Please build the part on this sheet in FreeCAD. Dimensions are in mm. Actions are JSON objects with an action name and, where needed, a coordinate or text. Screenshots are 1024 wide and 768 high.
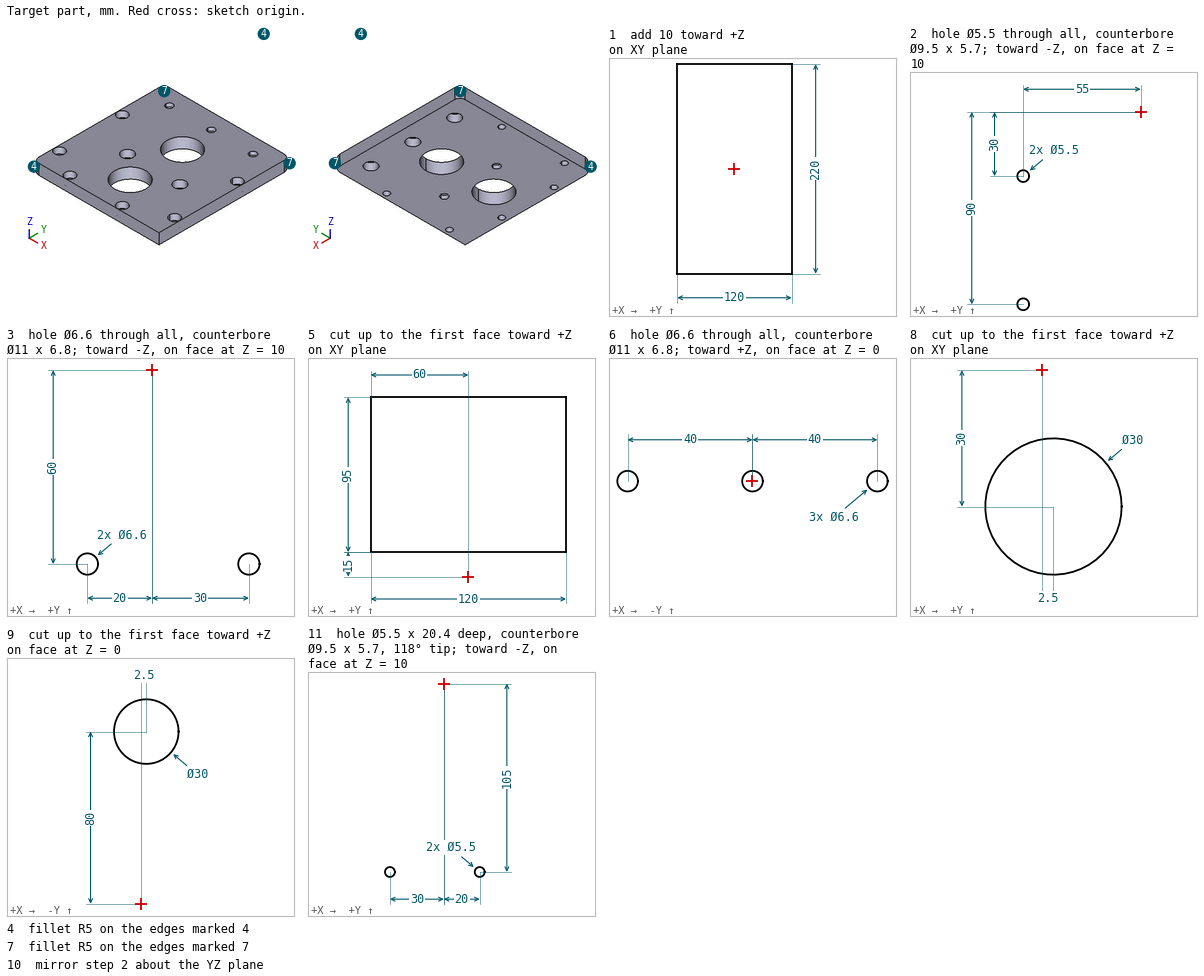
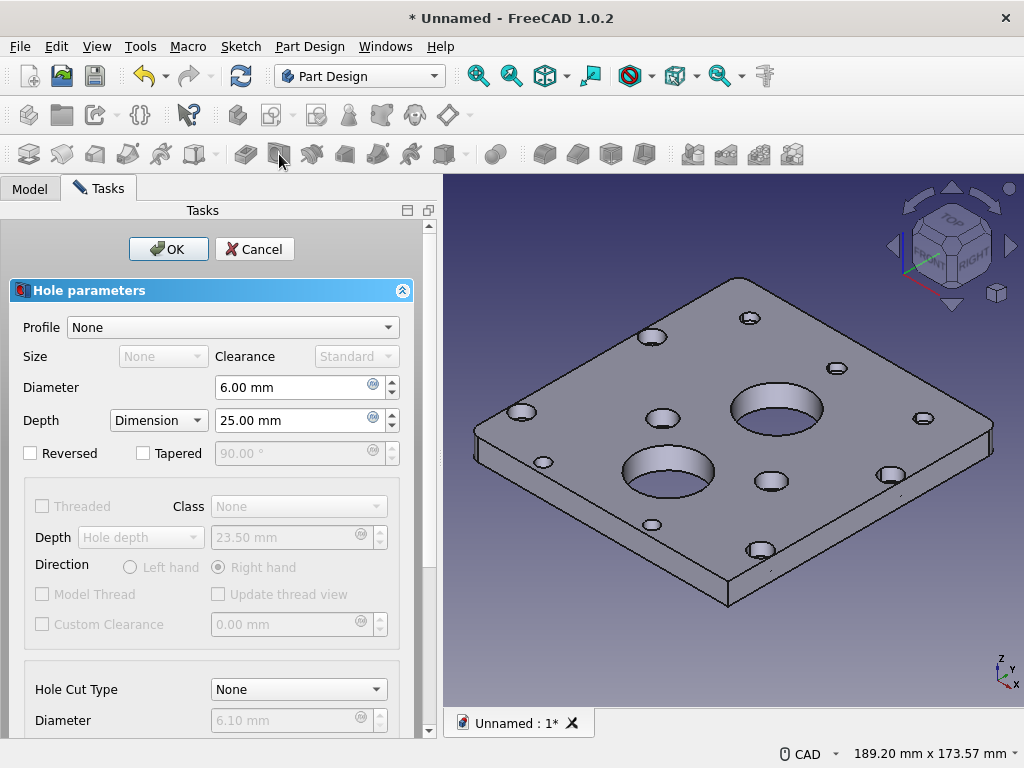
{"action": "triple_click", "coordinate": [300, 388]}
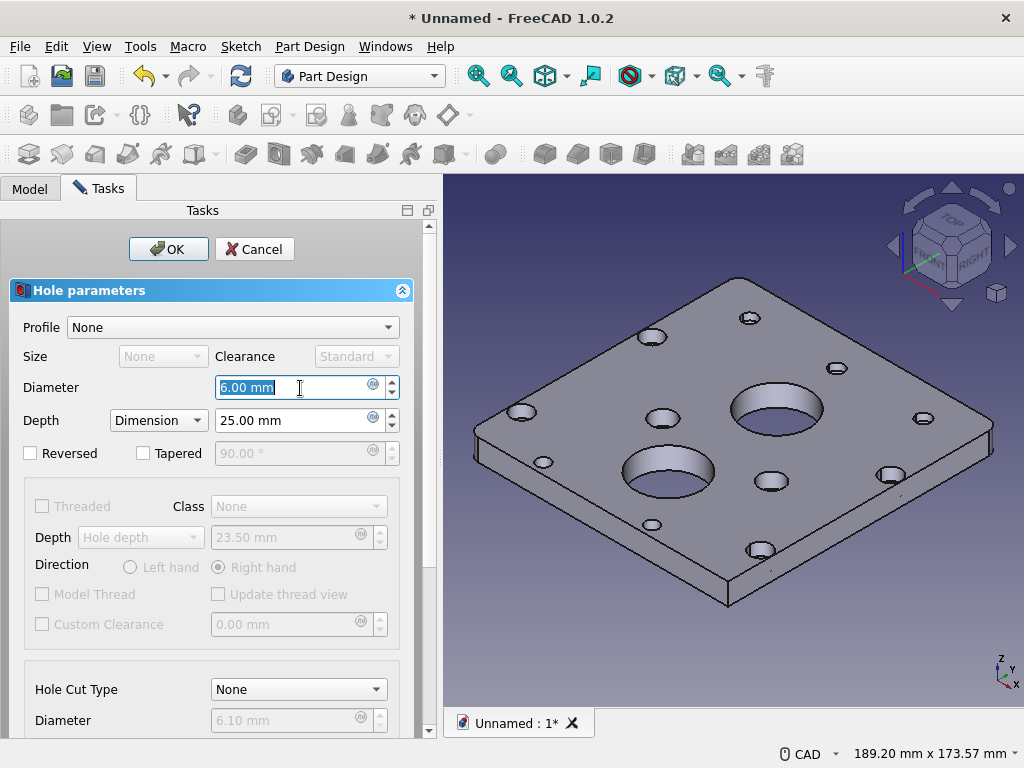
{"action": "type", "text": "5.5"}
{"action": "key", "text": "Tab"}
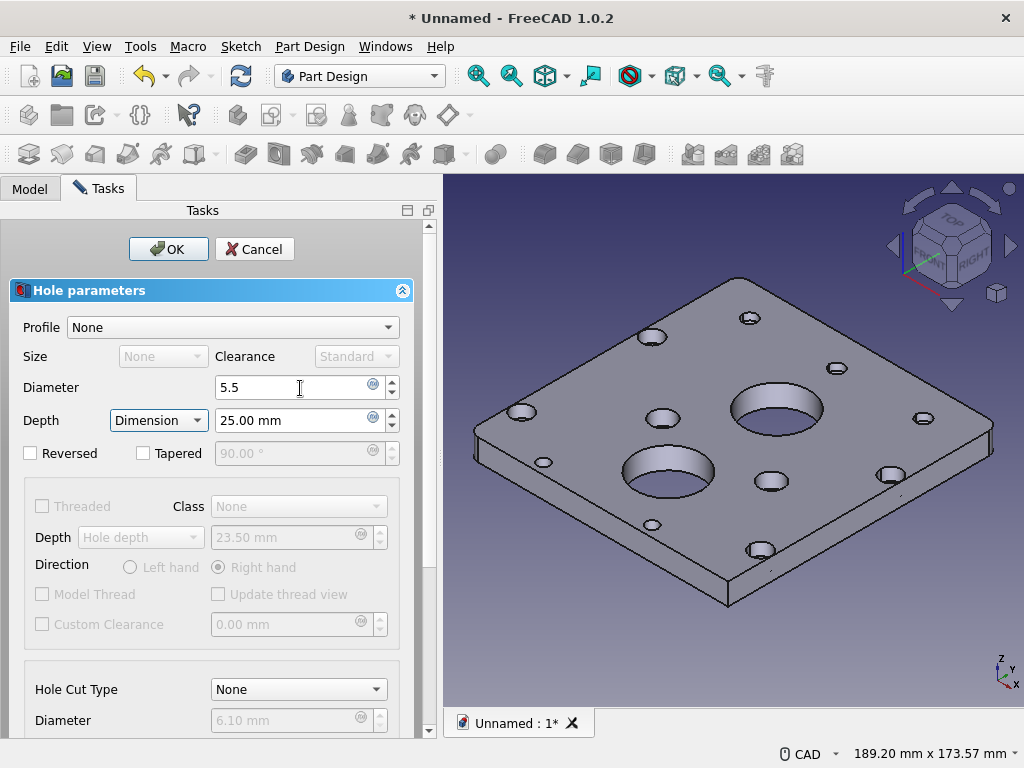
{"action": "triple_click", "coordinate": [300, 420]}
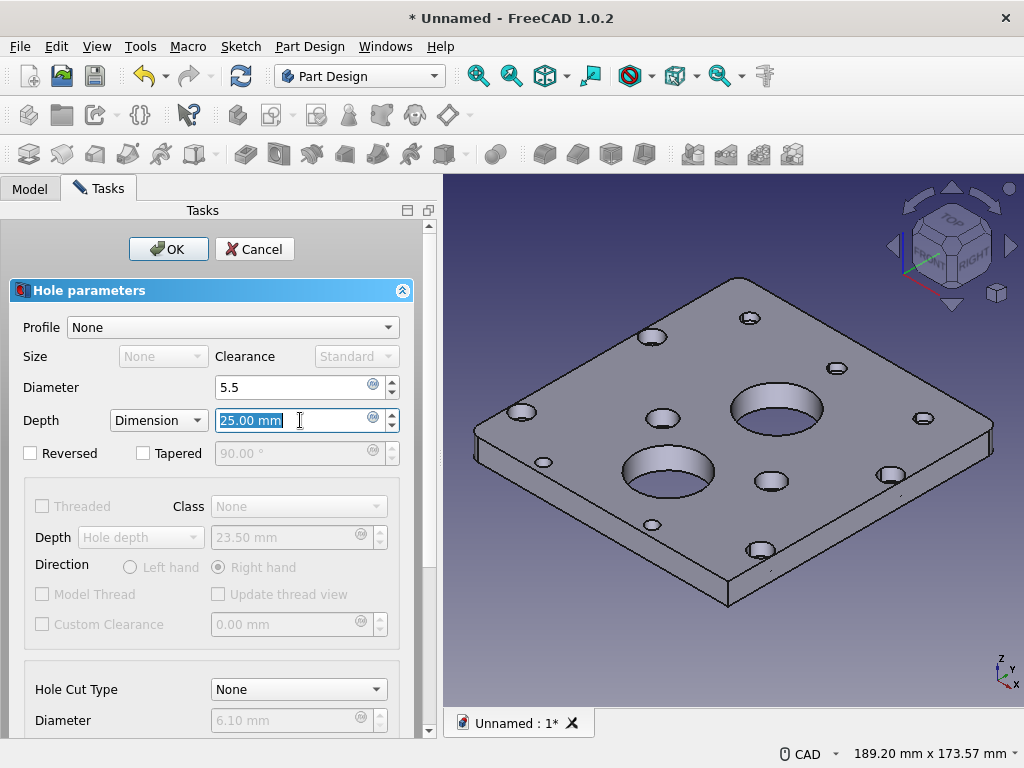
{"action": "type", "text": "20.4"}
{"action": "key", "text": "Tab"}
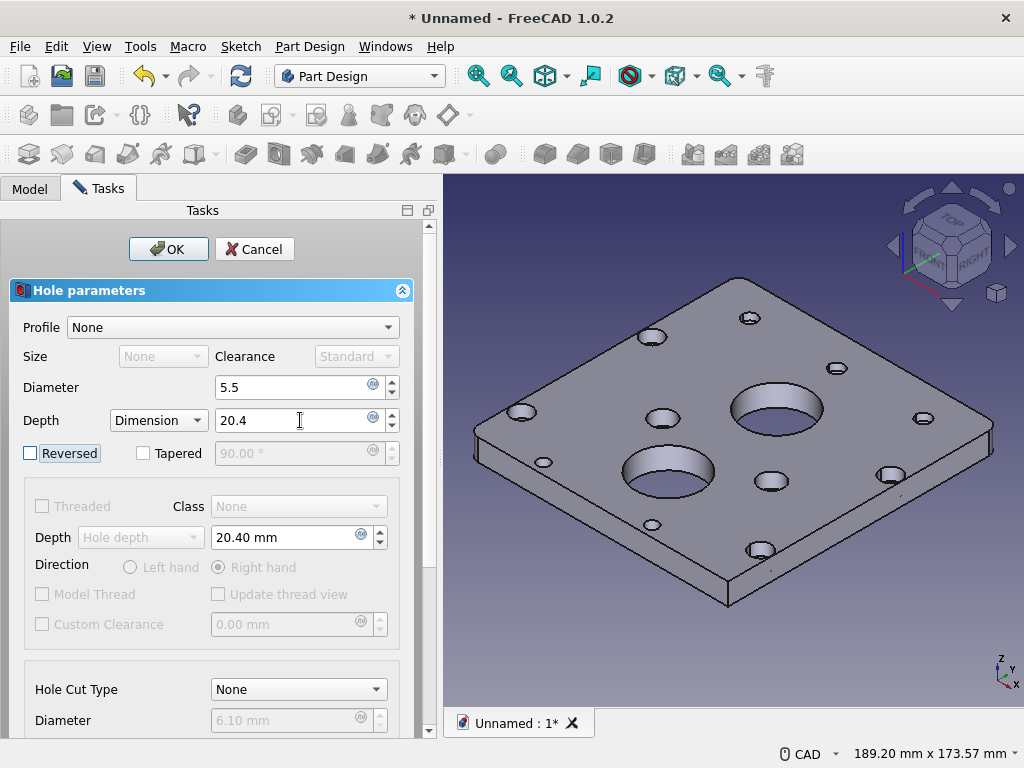
{"action": "left_click", "coordinate": [300, 690]}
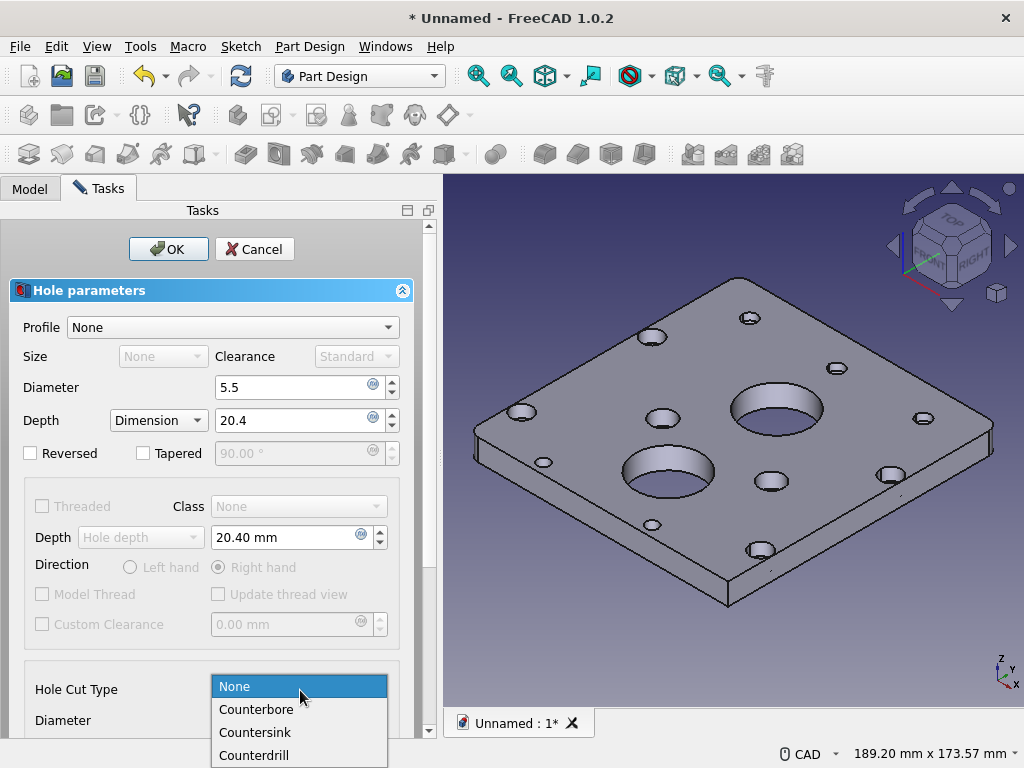
{"action": "left_click", "coordinate": [298, 710]}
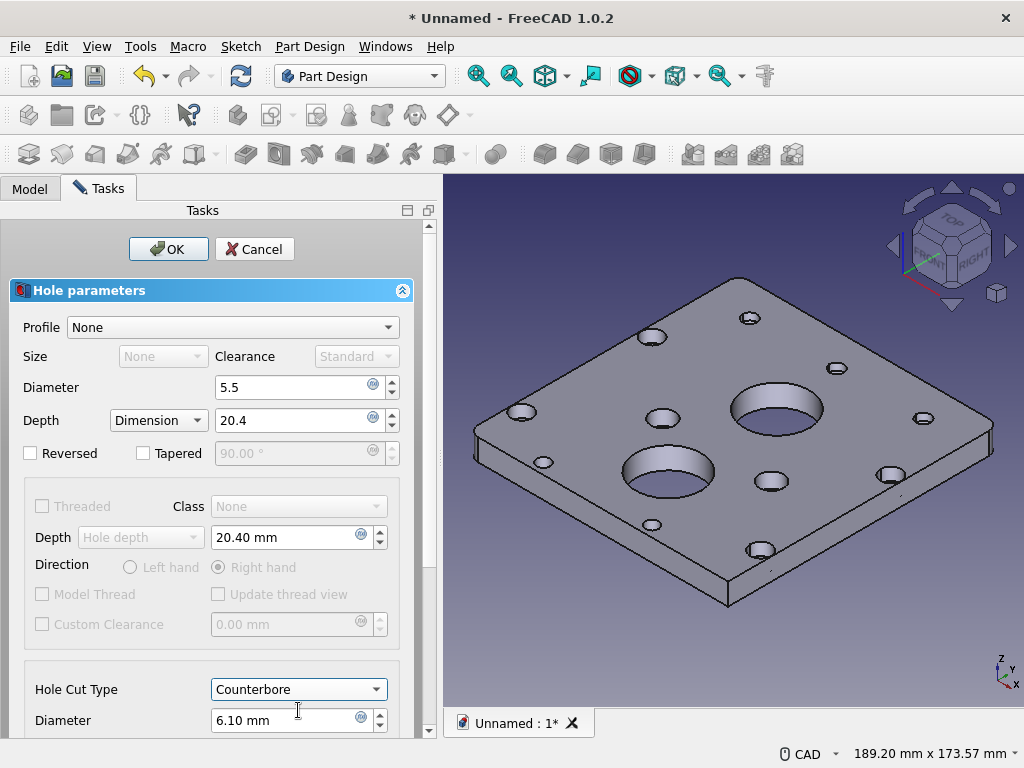
{"action": "triple_click", "coordinate": [292, 720]}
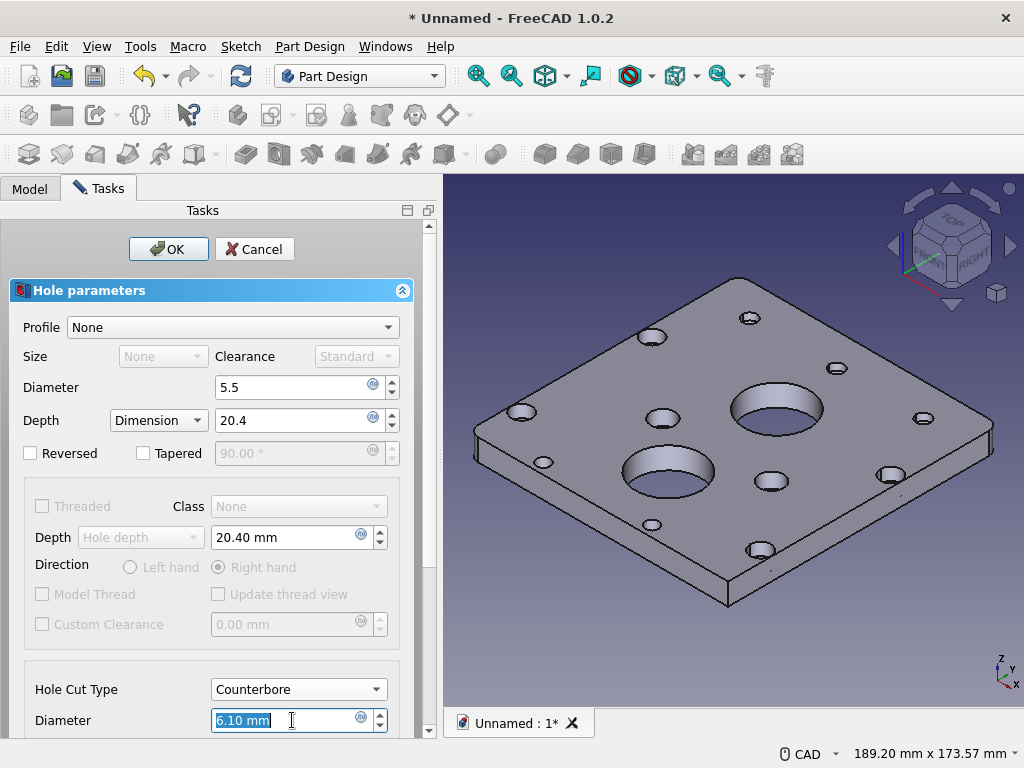
{"action": "type", "text": "9.5"}
{"action": "key", "text": "Tab"}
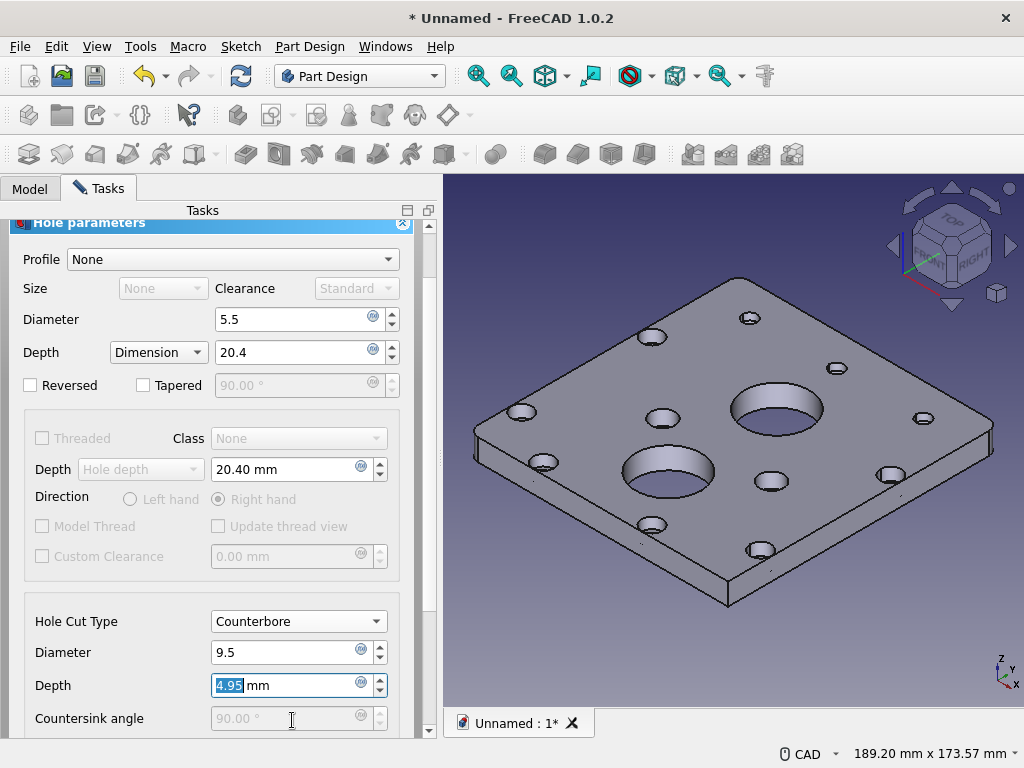
{"action": "type", "text": "5.7"}
{"action": "key", "text": "Tab"}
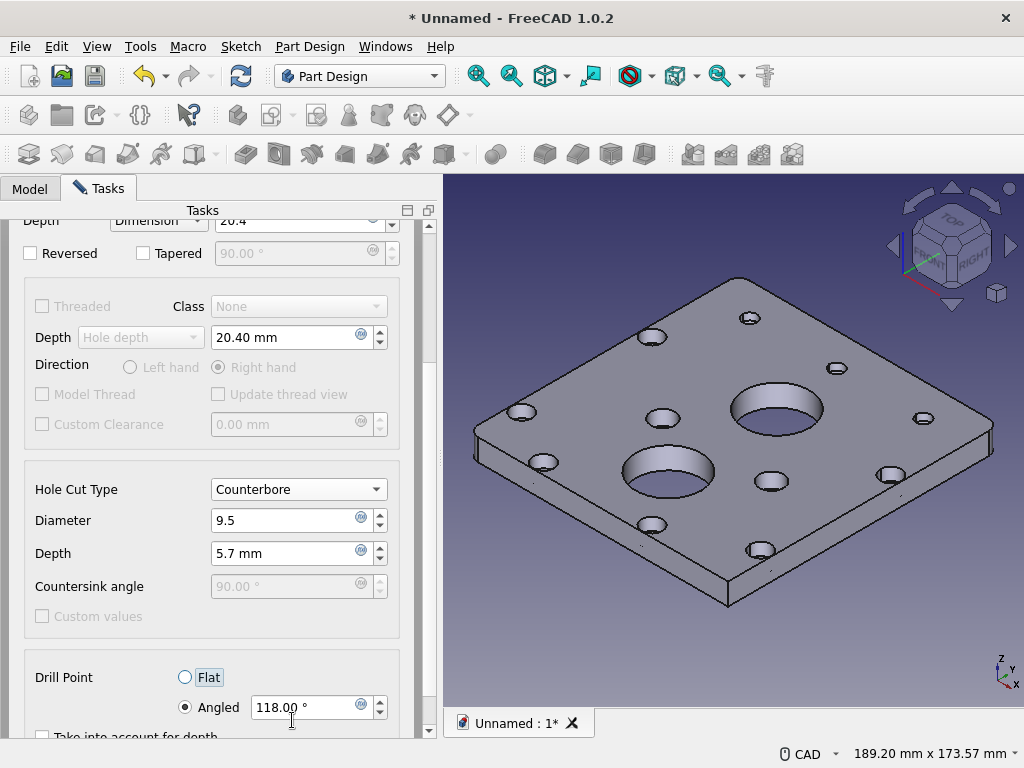
{"action": "scroll", "coordinate": [429, 479], "scroll_direction": "up", "scroll_amount": 5}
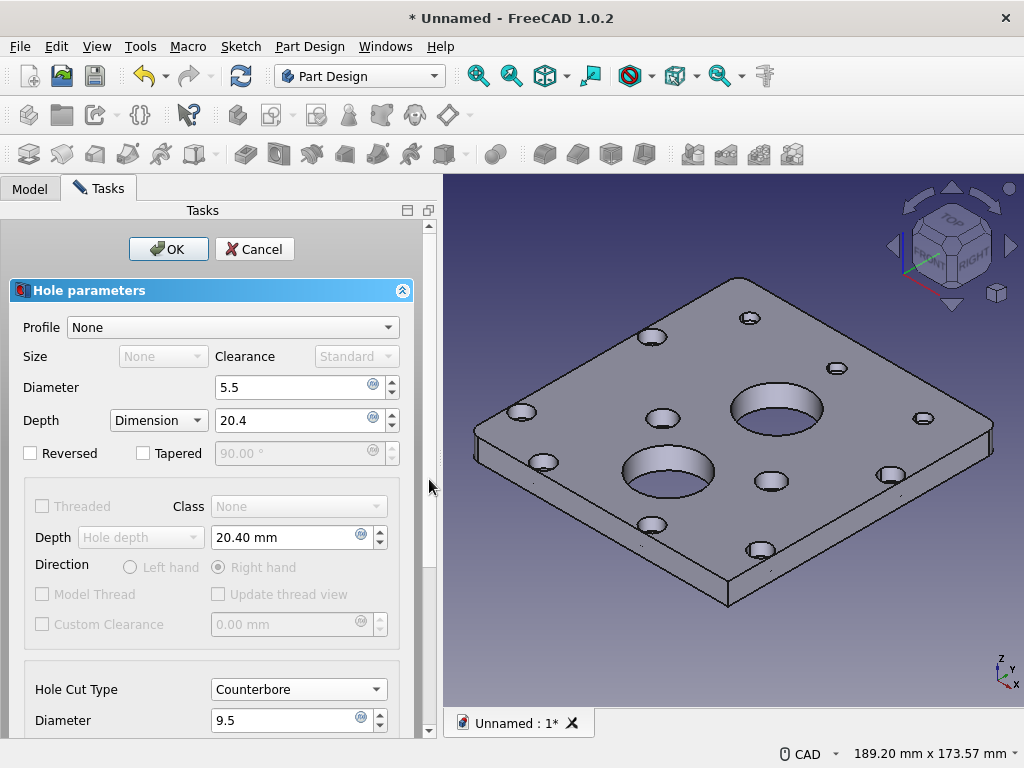
{"action": "left_click", "coordinate": [169, 249]}